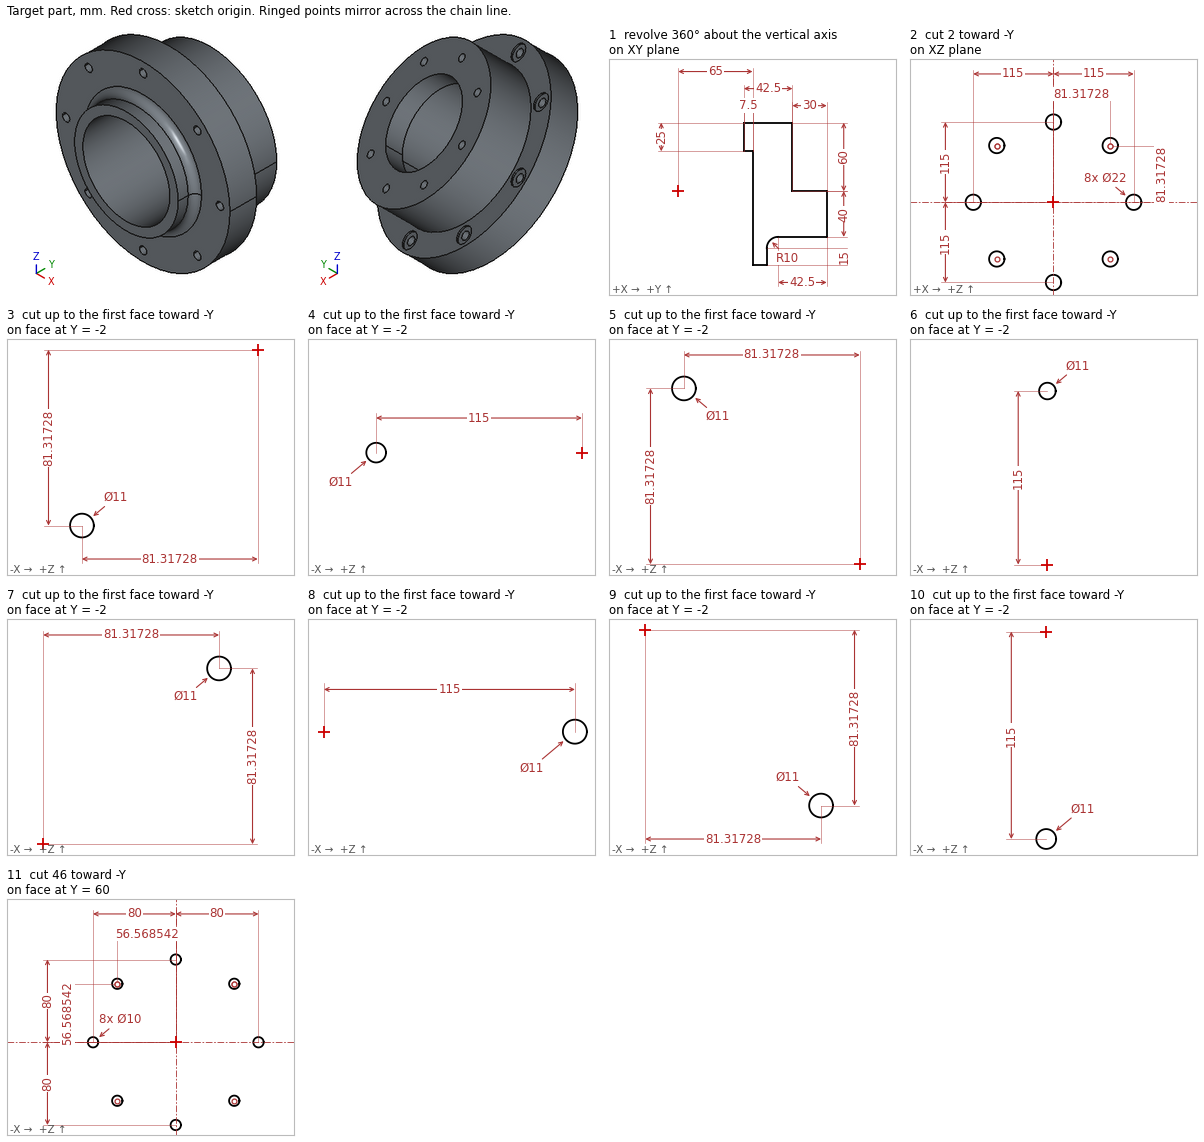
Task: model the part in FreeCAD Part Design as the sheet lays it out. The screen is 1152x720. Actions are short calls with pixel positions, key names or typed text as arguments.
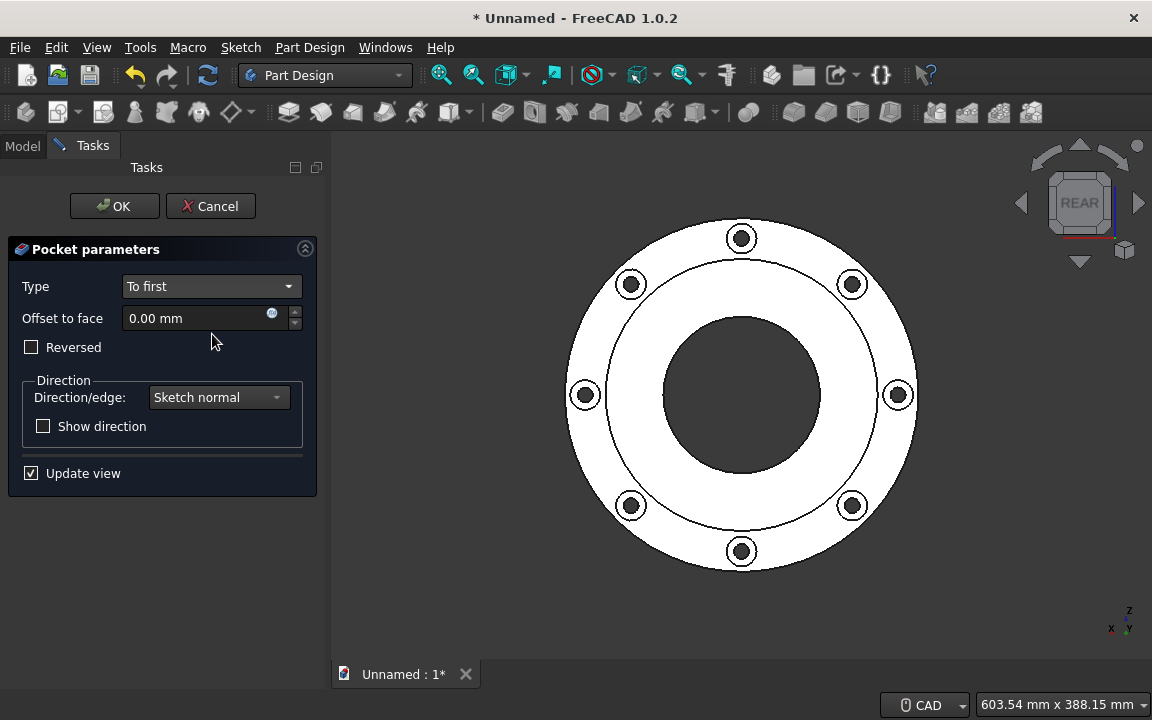
click(115, 206)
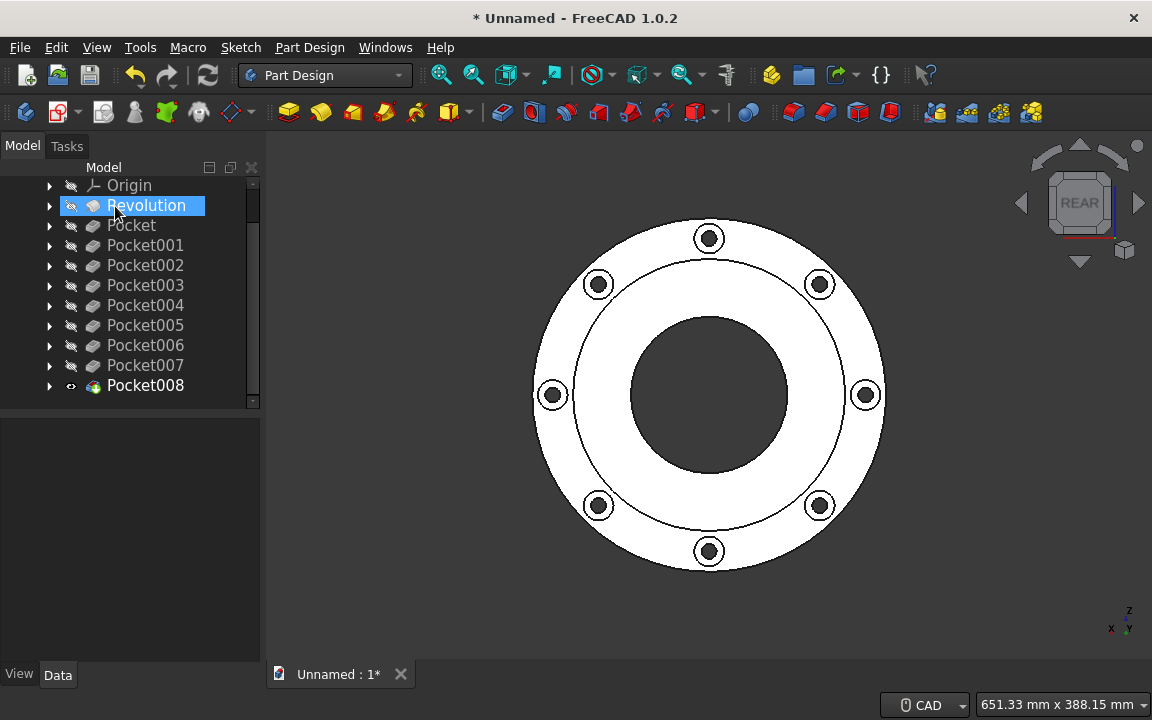
click(631, 472)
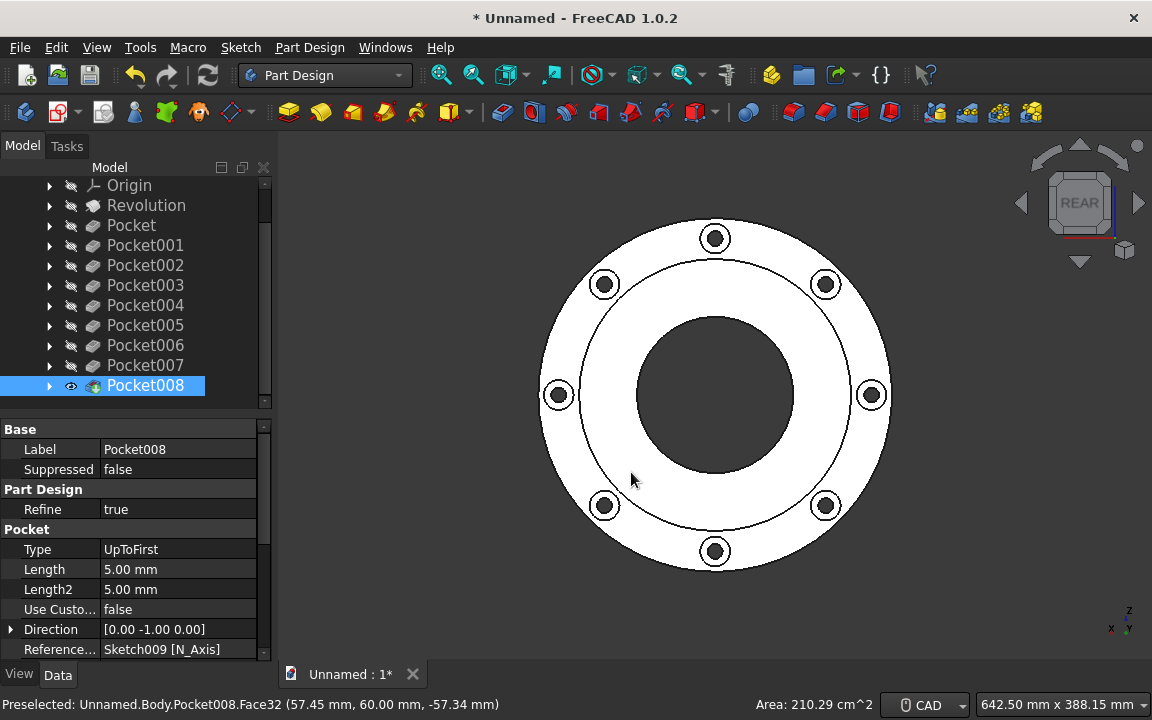
click(58, 112)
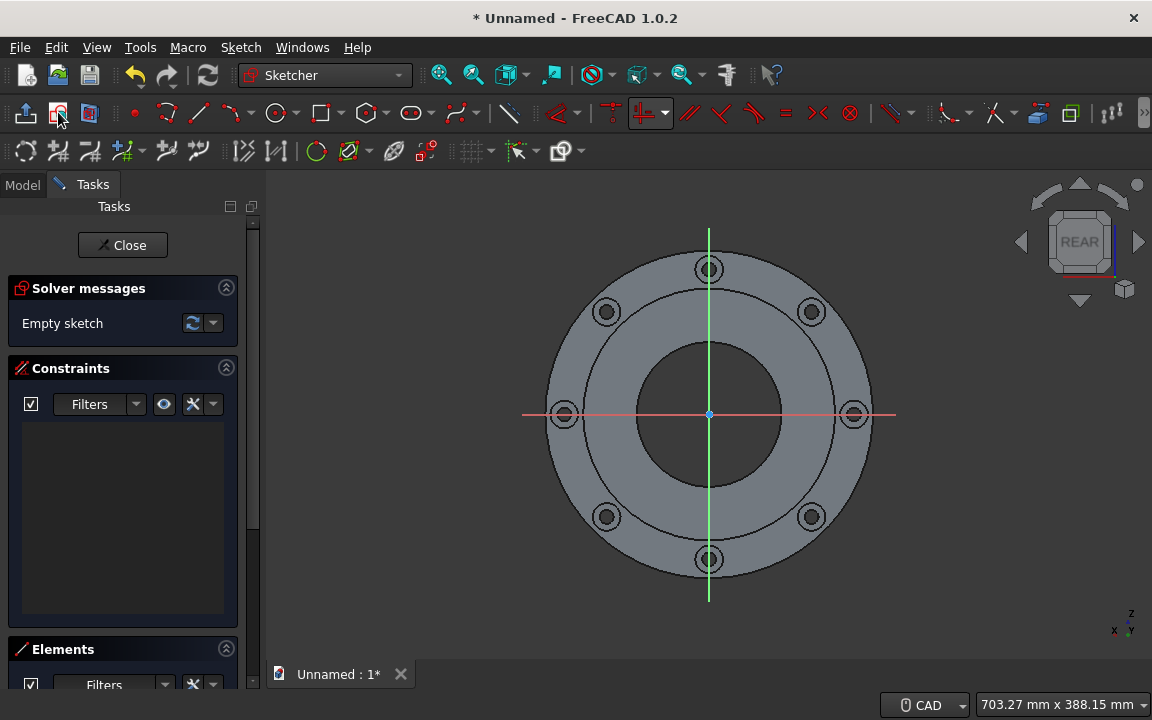
scroll(849, 415, up, 2)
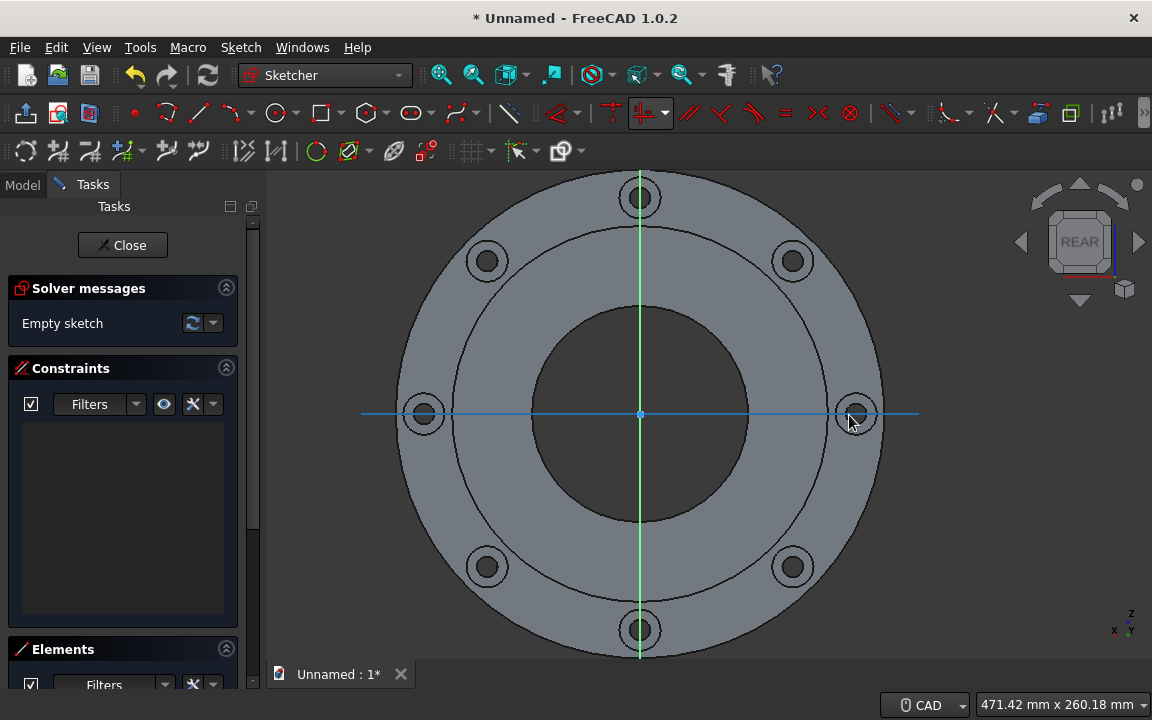
click(276, 114)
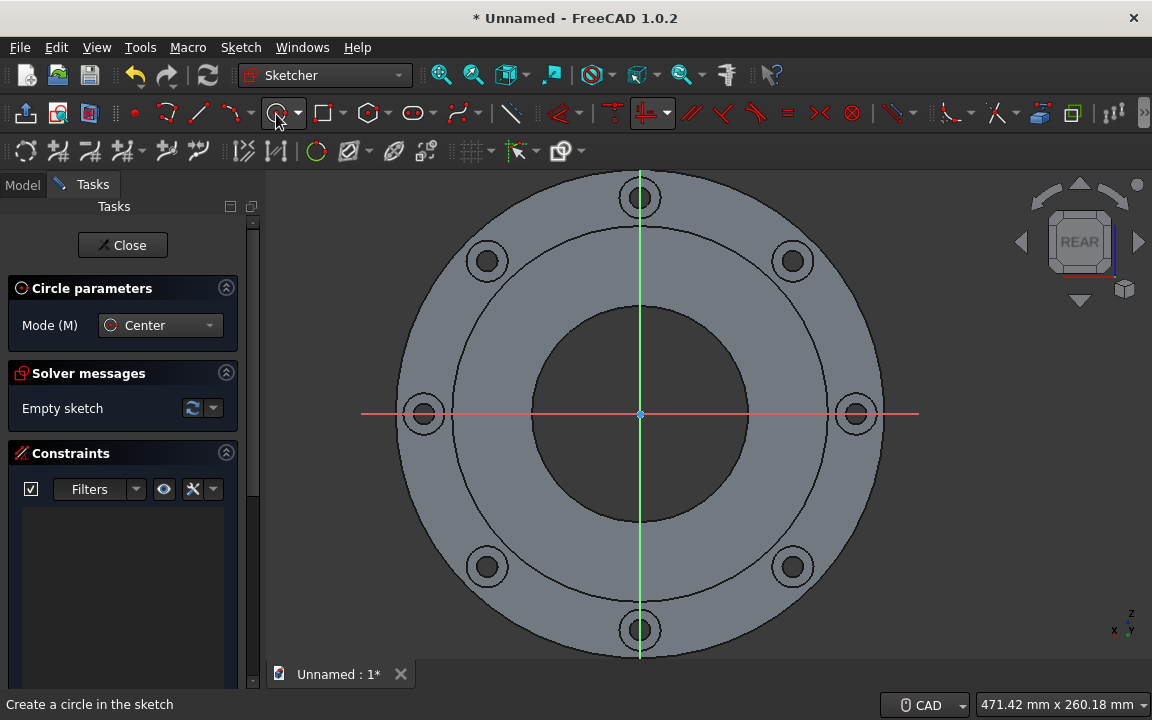
scroll(490, 414, up, 5)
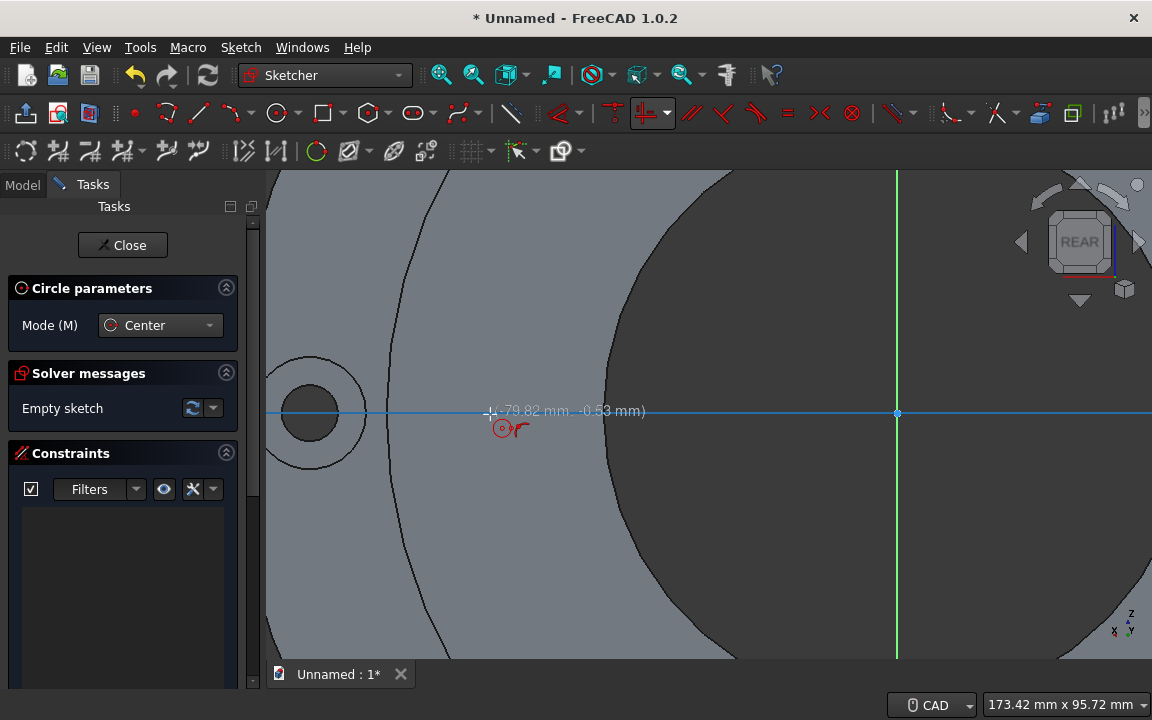
click(489, 413)
move(507, 395)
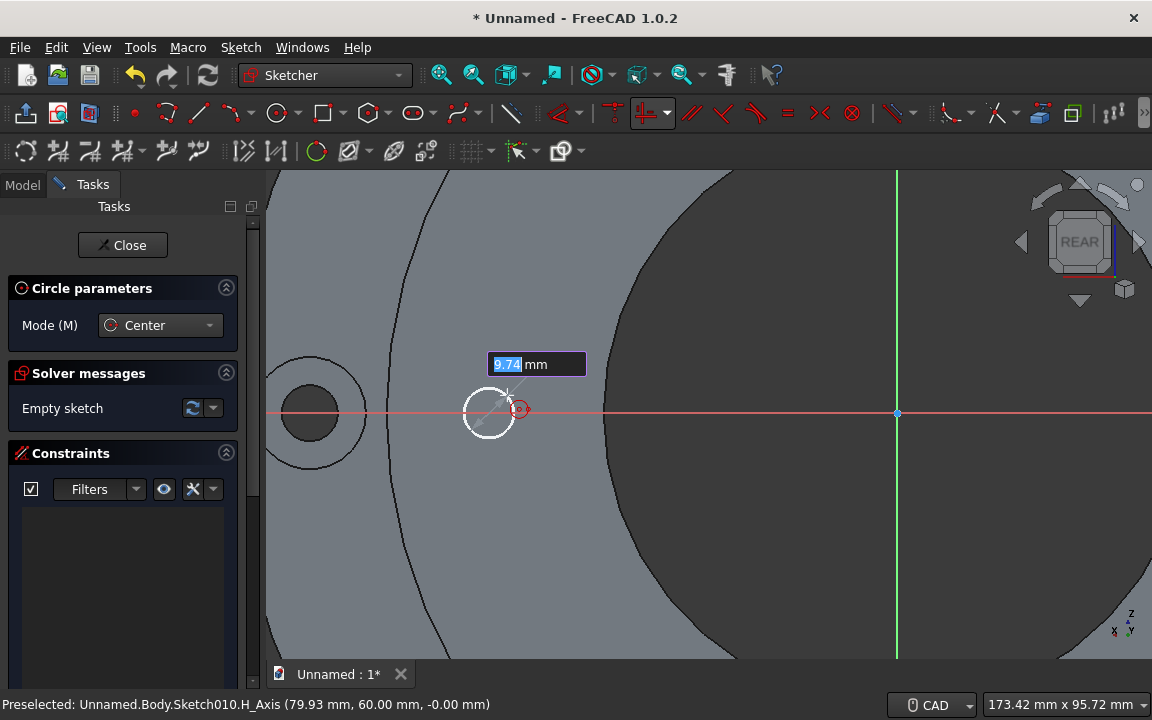
text(10)
key(Return)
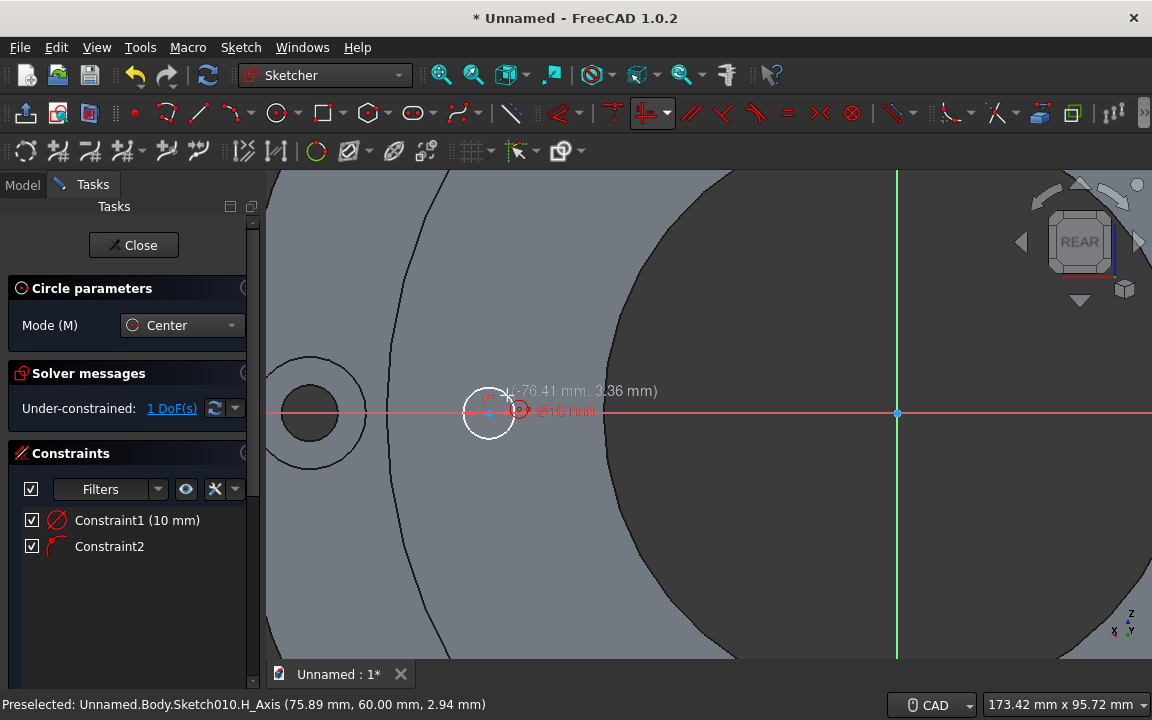
scroll(491, 415, down, 5)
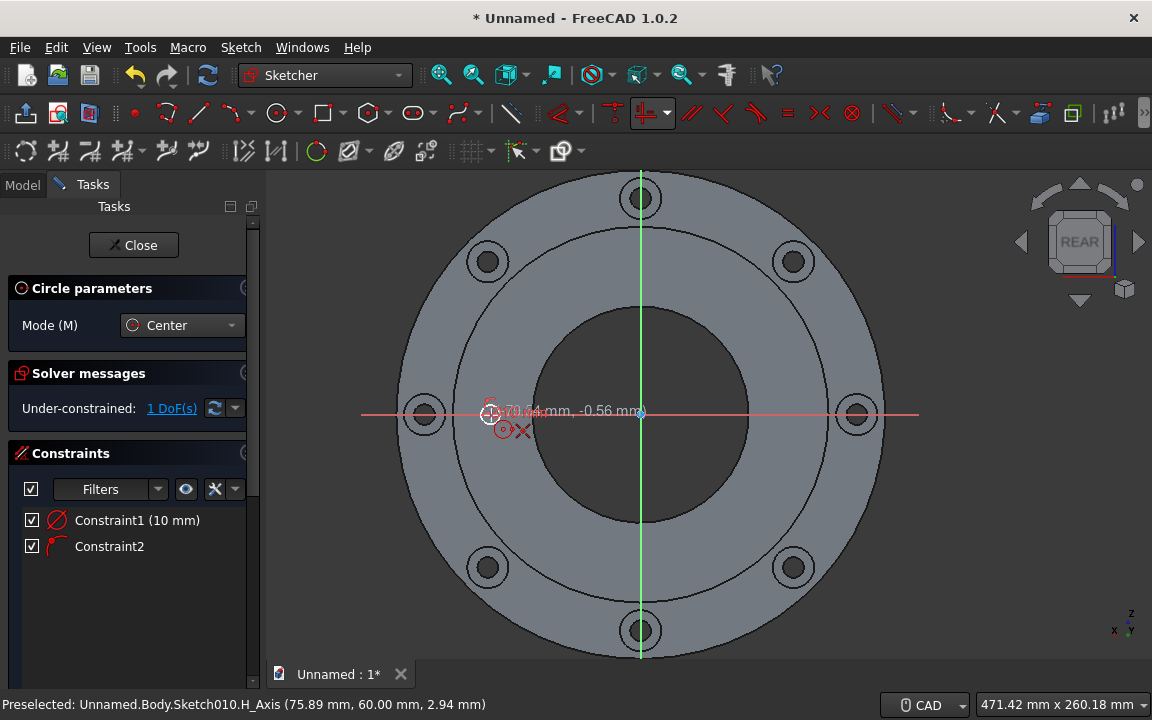
scroll(534, 308, up, 5)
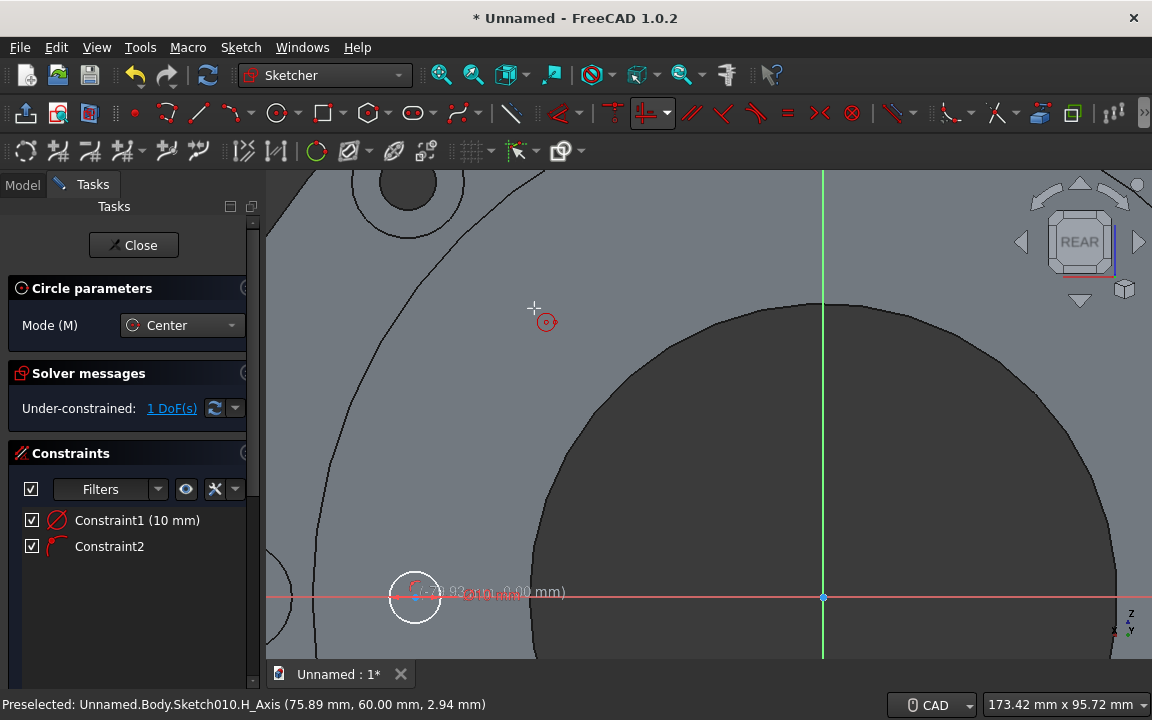
click(534, 308)
move(552, 290)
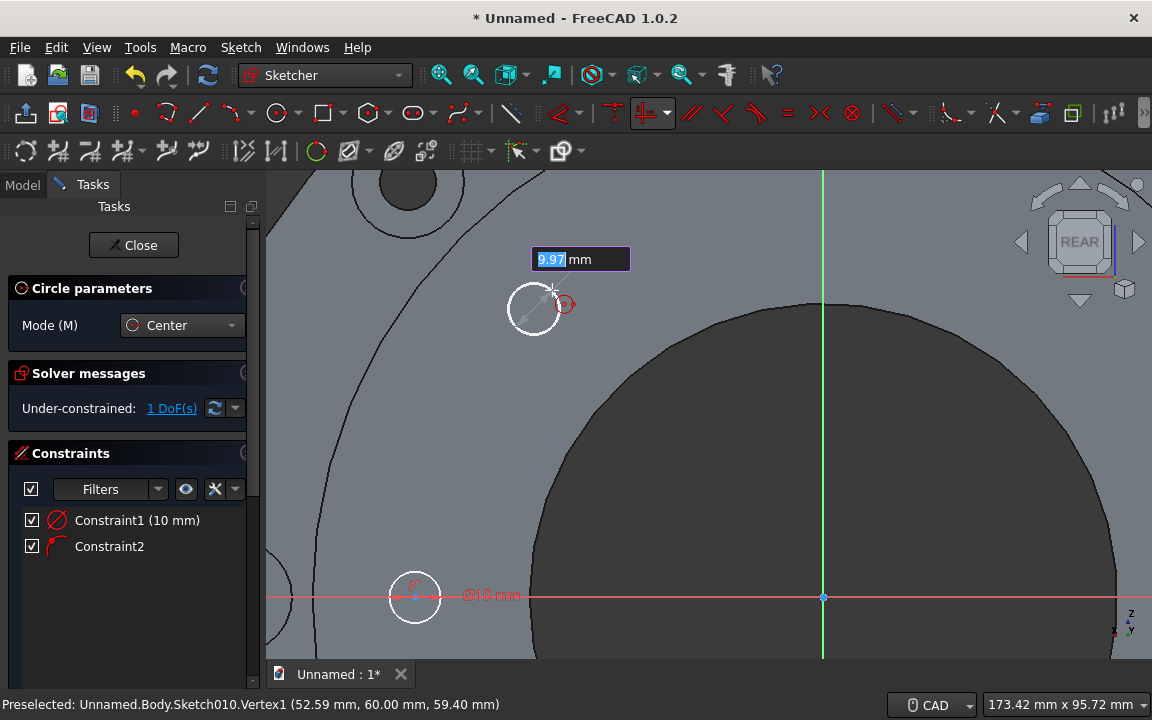
text(10)
key(Return)